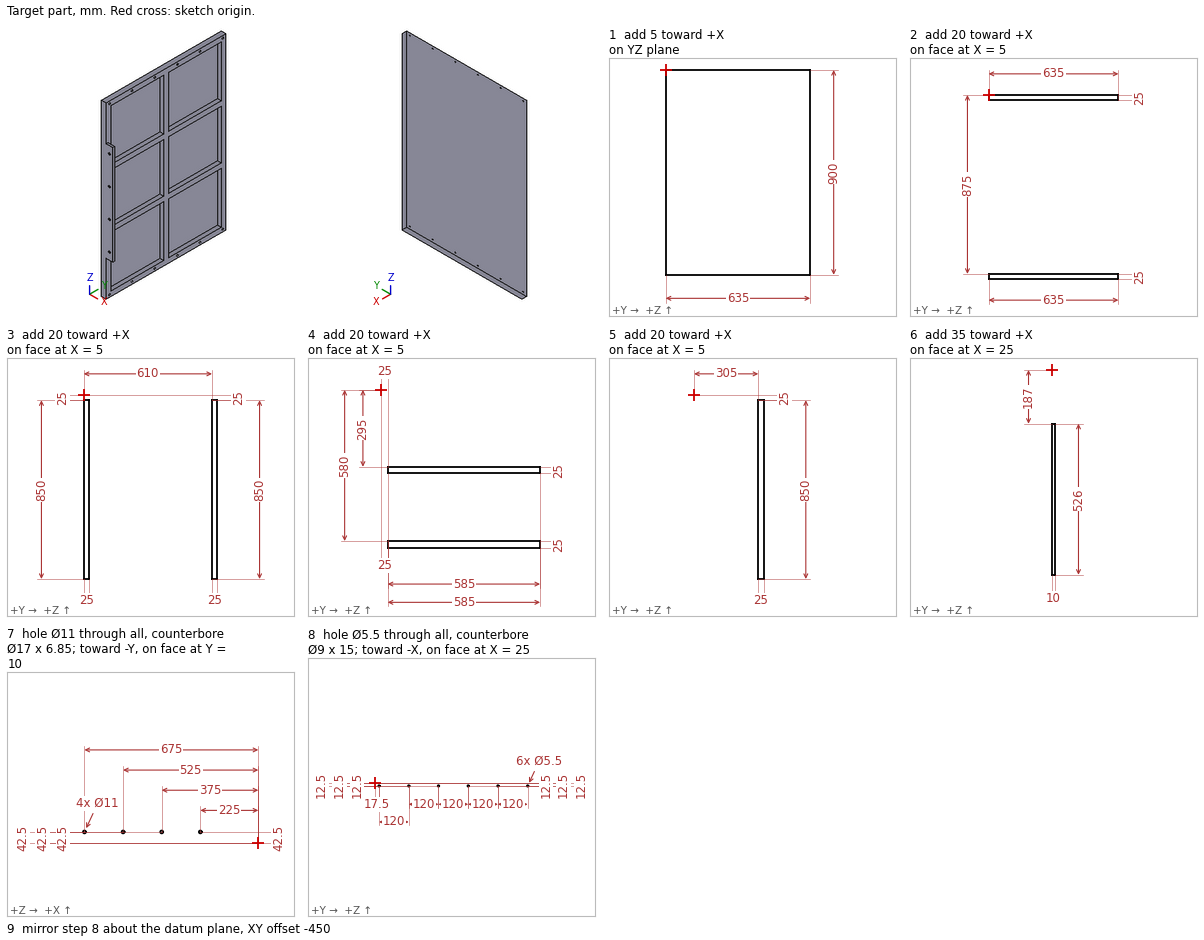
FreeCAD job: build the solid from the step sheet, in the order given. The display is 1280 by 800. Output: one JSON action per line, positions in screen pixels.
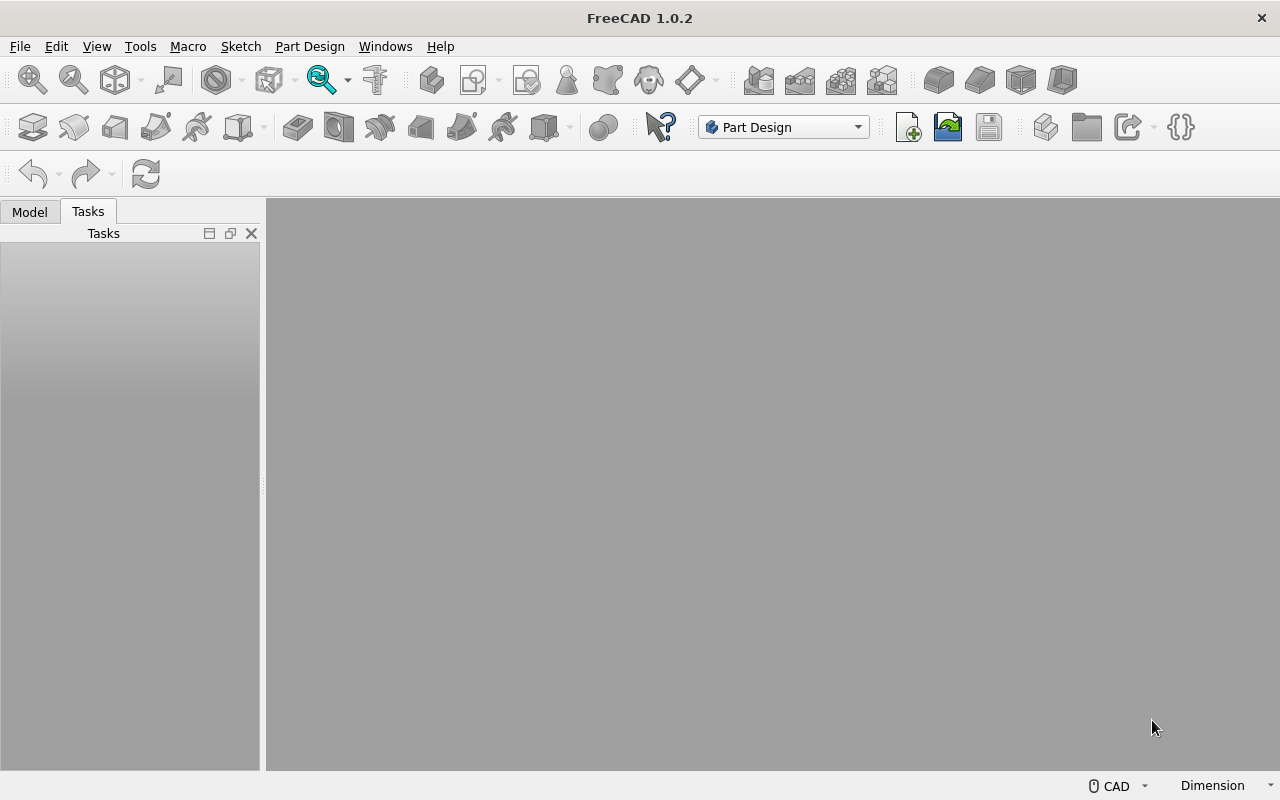
{"action": "left_click", "coordinate": [907, 128]}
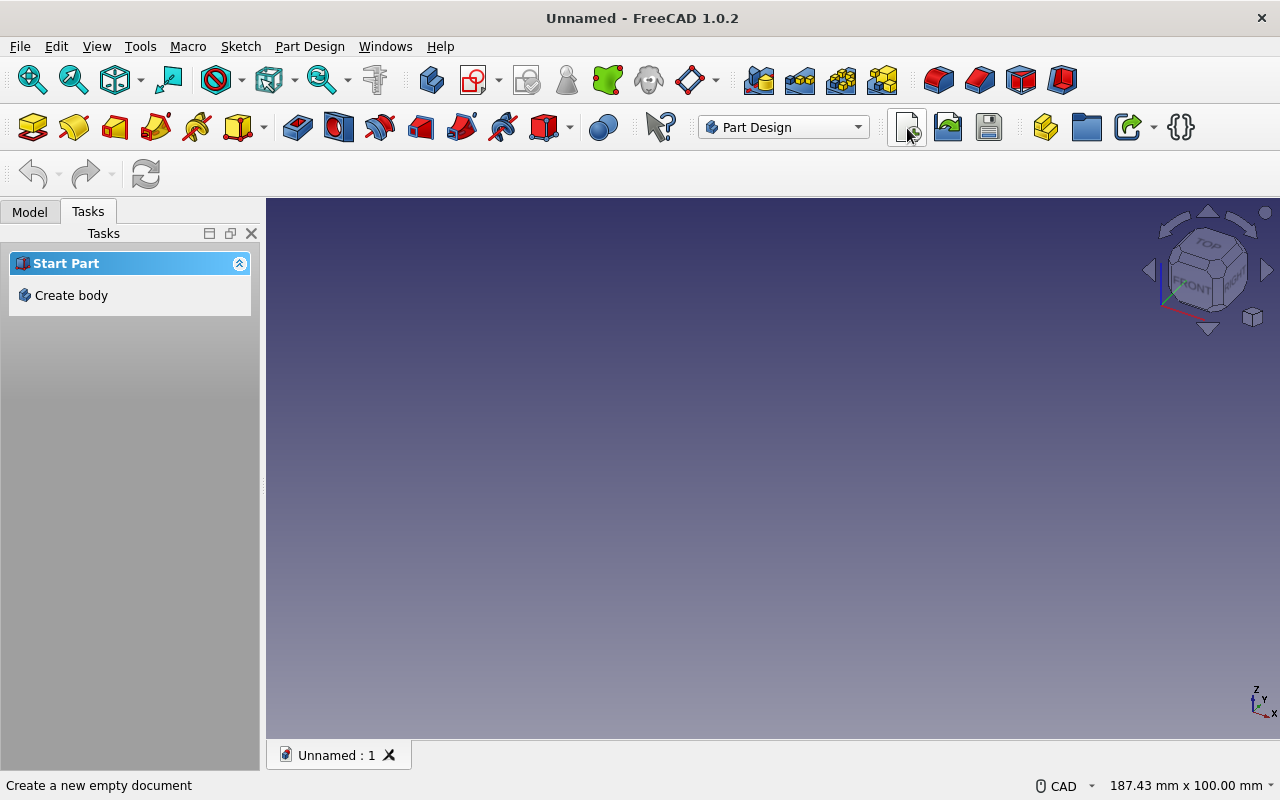
{"action": "left_click", "coordinate": [472, 80]}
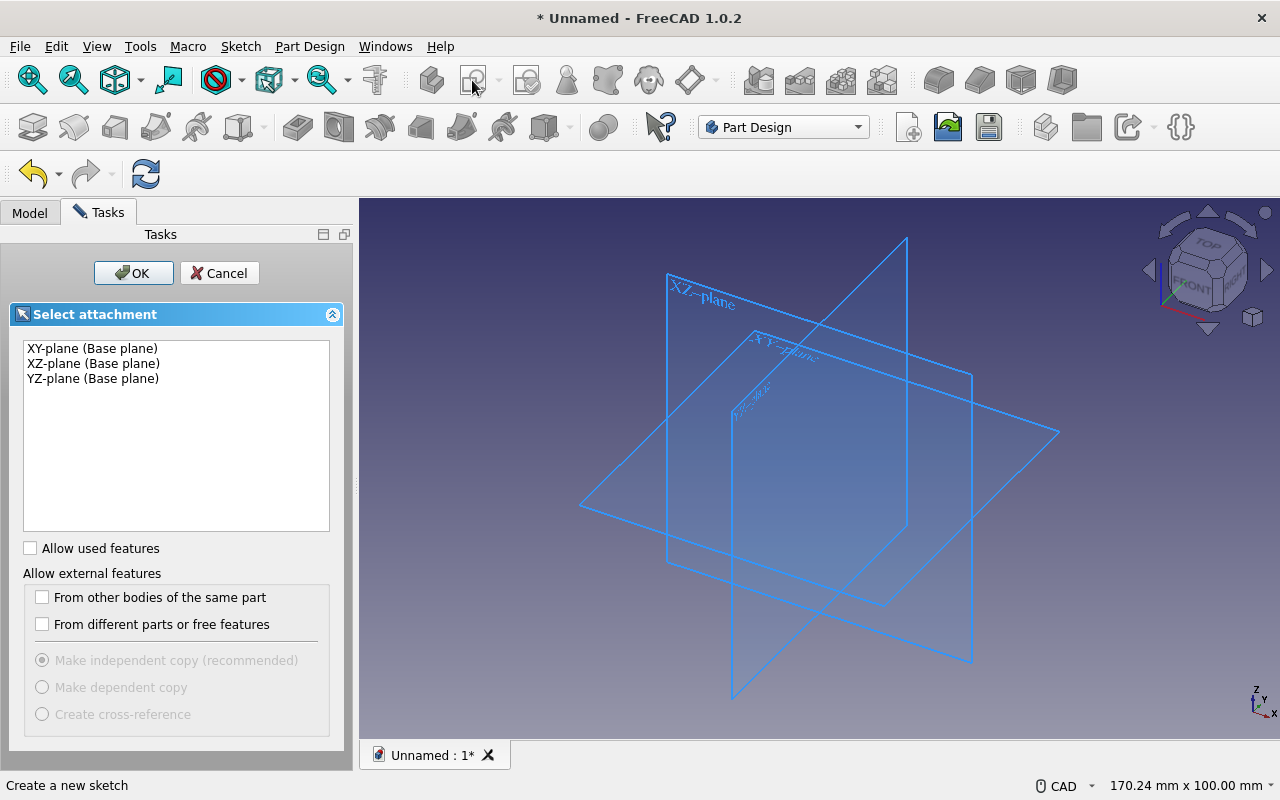
{"action": "left_click", "coordinate": [84, 378]}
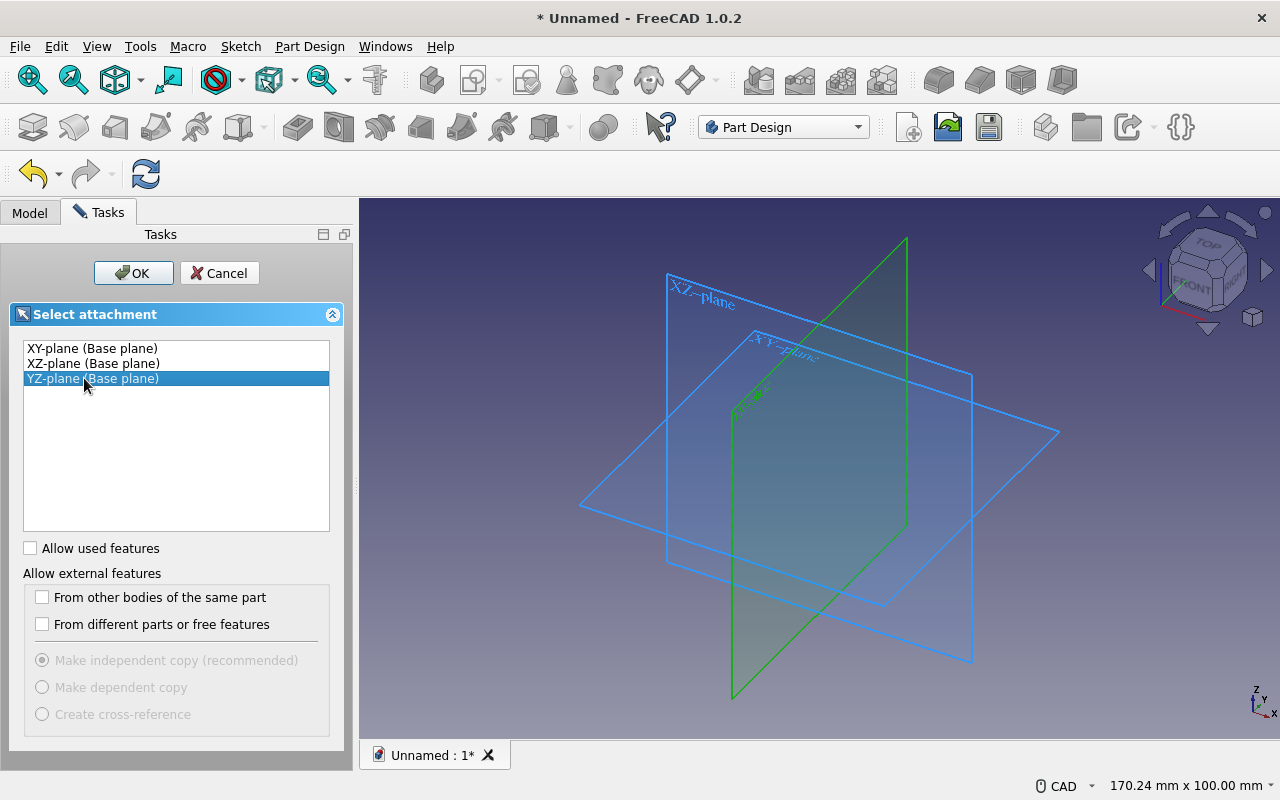
{"action": "left_click", "coordinate": [134, 273]}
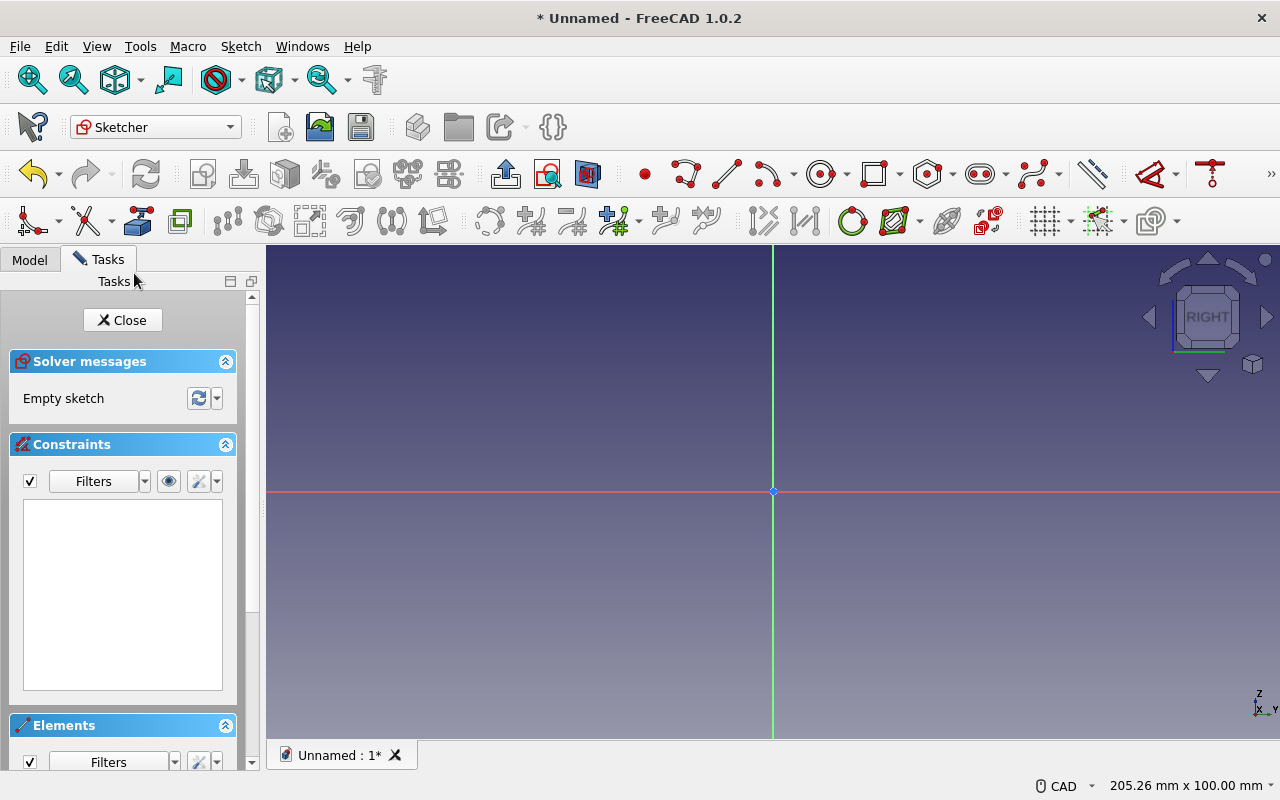
{"action": "scroll", "coordinate": [573, 314], "scroll_direction": "down", "scroll_amount": 13}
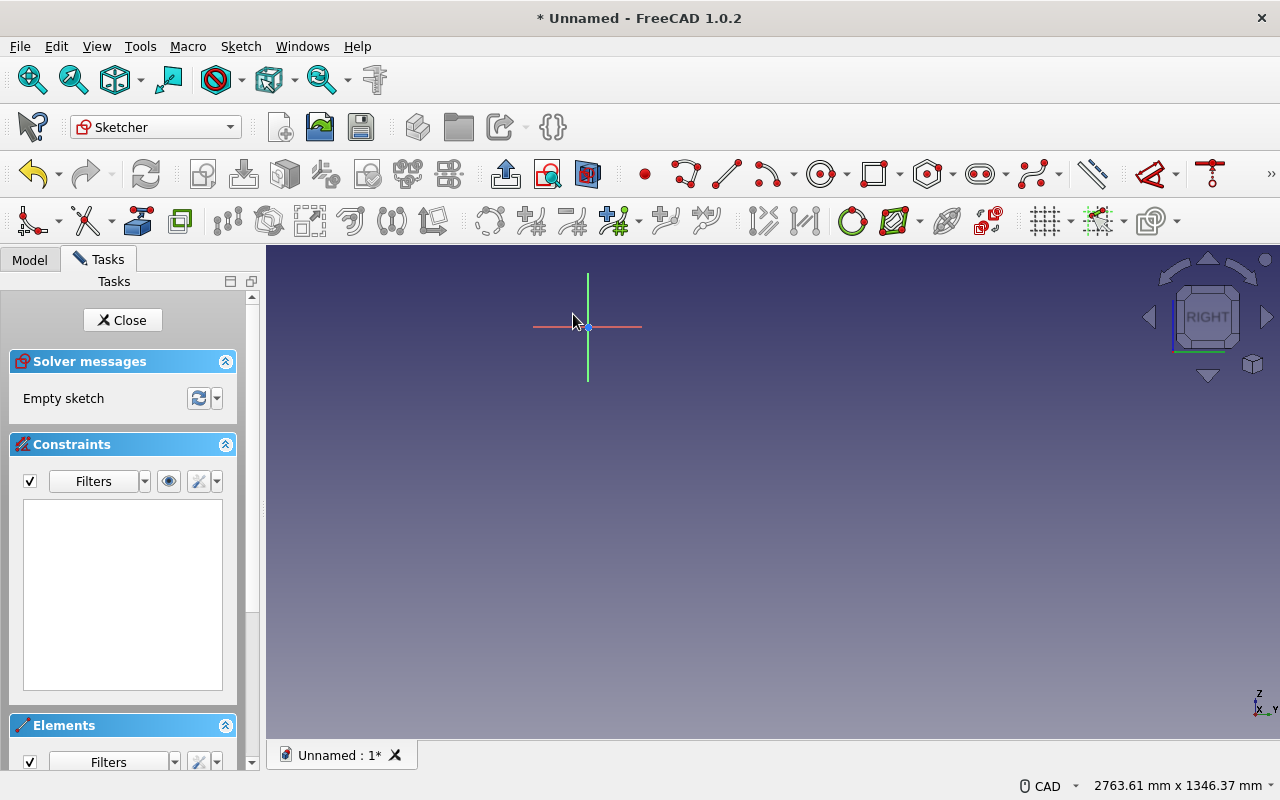
{"action": "left_click", "coordinate": [874, 174]}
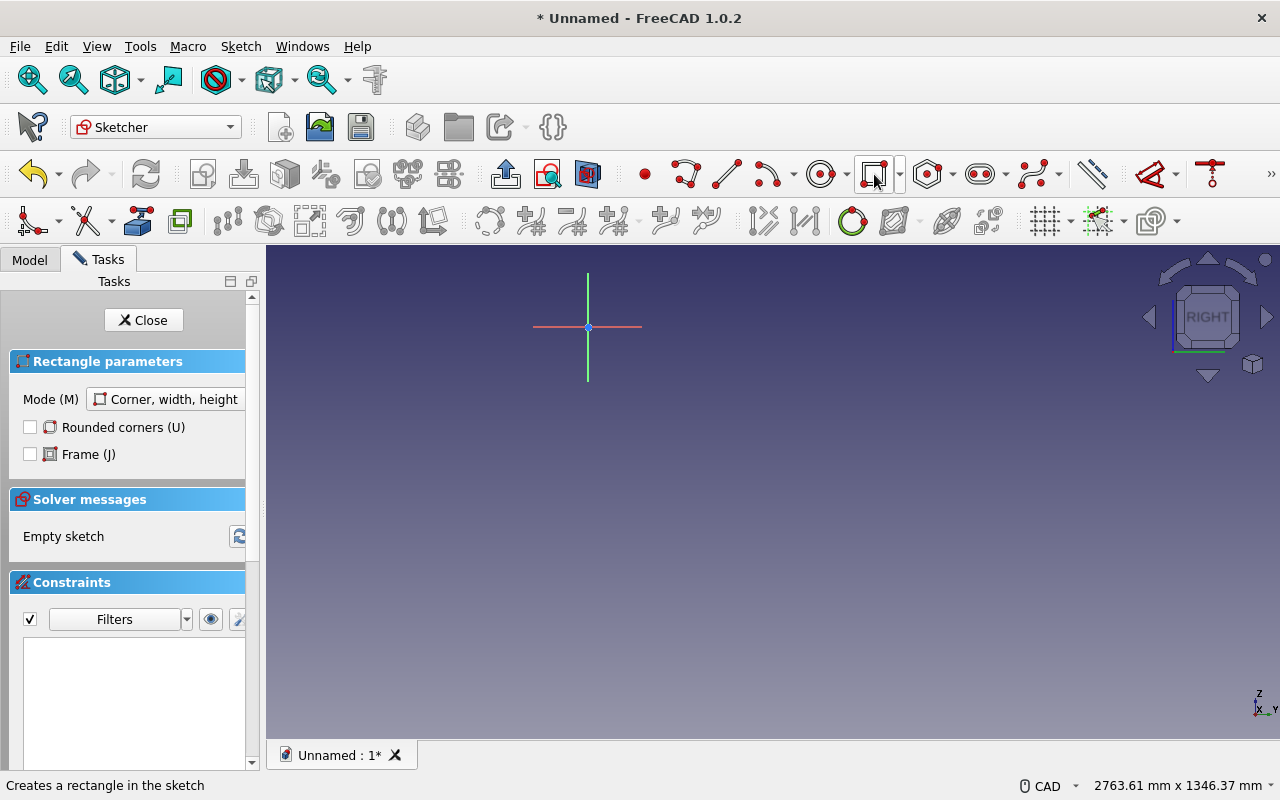
{"action": "left_click", "coordinate": [588, 327]}
{"action": "mouse_move", "coordinate": [821, 658]}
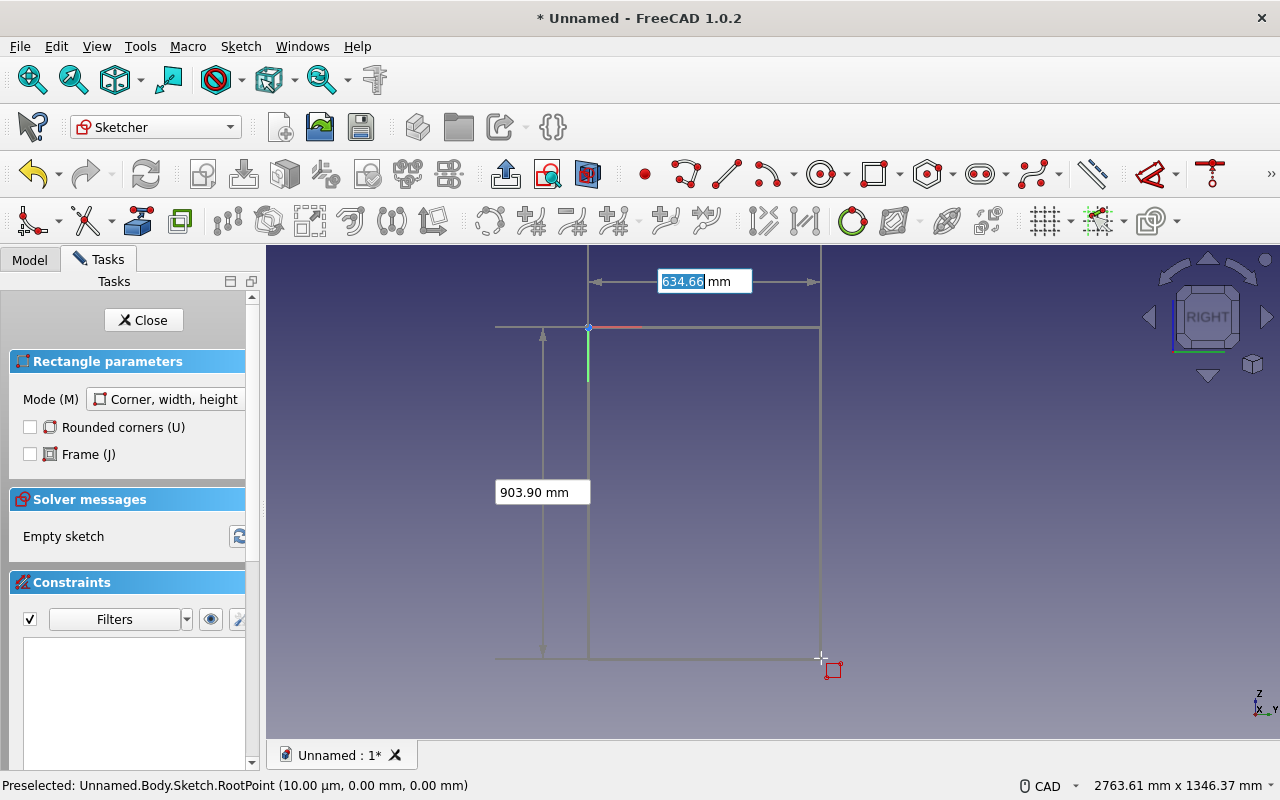
{"action": "type", "text": "635"}
{"action": "key", "text": "Tab"}
{"action": "type", "text": "900"}
{"action": "key", "text": "Return"}
{"action": "key", "text": "Escape"}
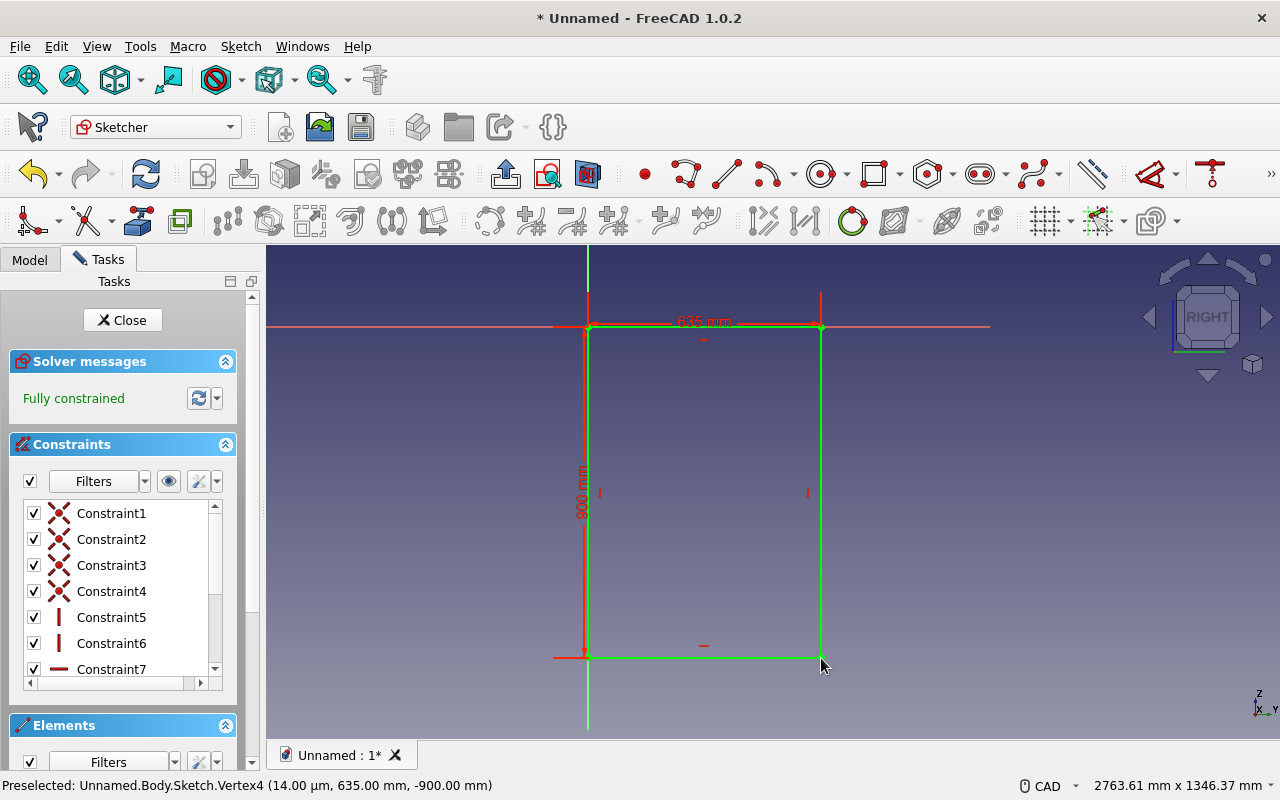
{"action": "left_click", "coordinate": [123, 320]}